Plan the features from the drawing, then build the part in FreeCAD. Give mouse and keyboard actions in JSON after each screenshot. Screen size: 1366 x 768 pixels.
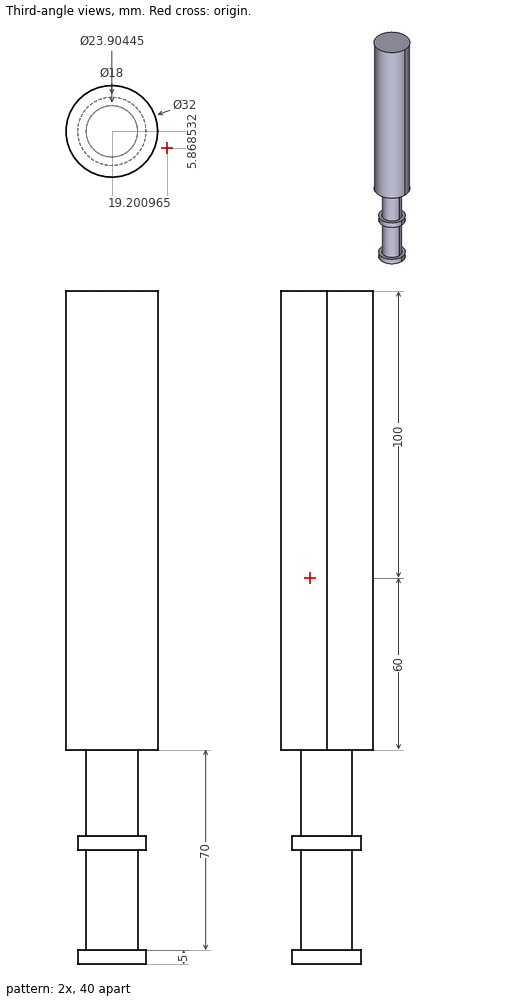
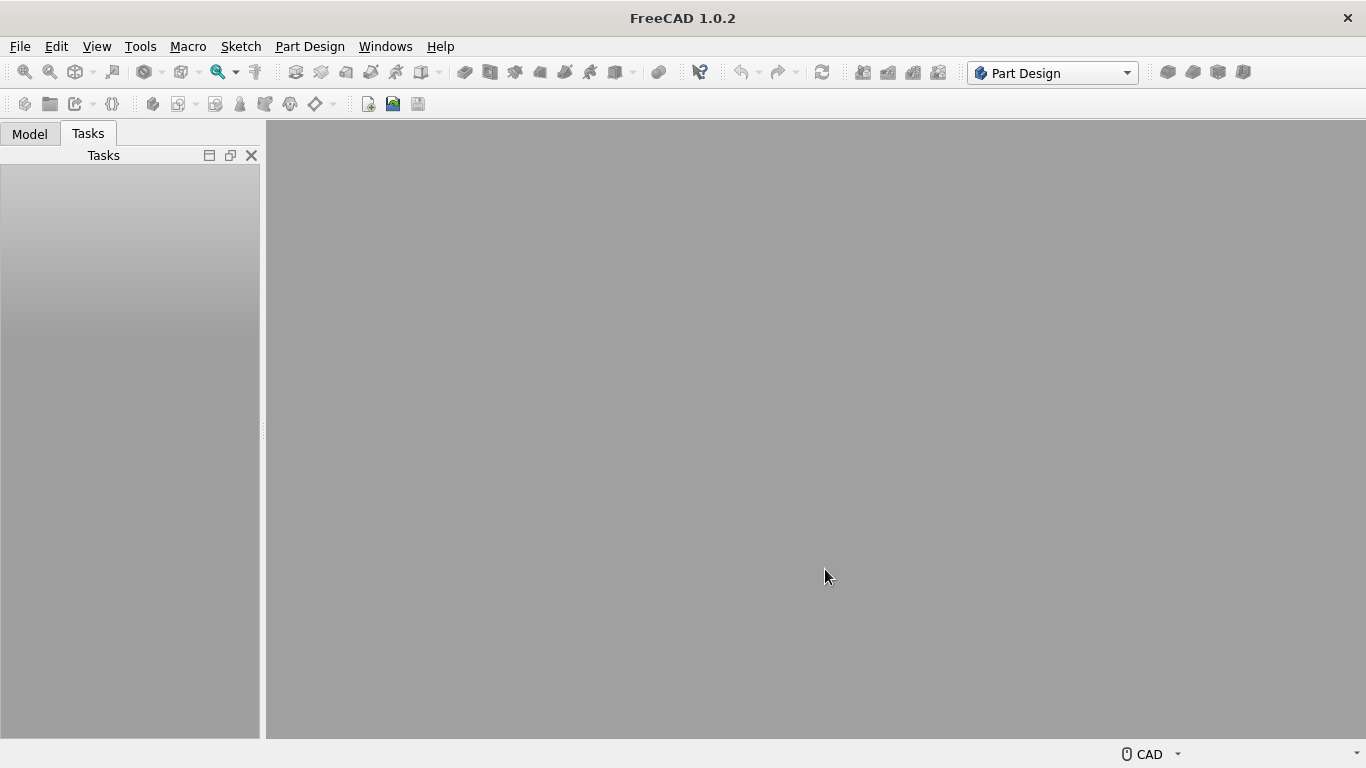
{"action": "key", "text": "ctrl+n"}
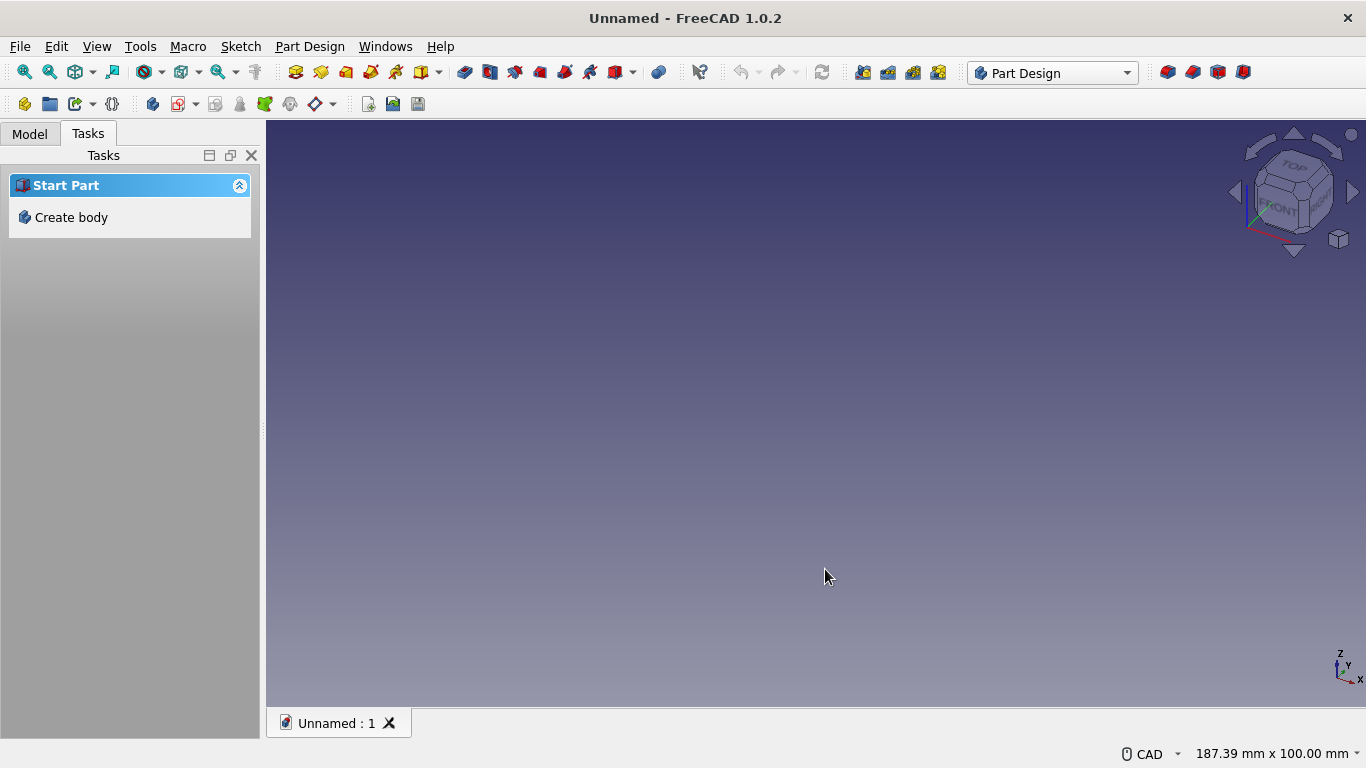
{"action": "left_click", "coordinate": [178, 104]}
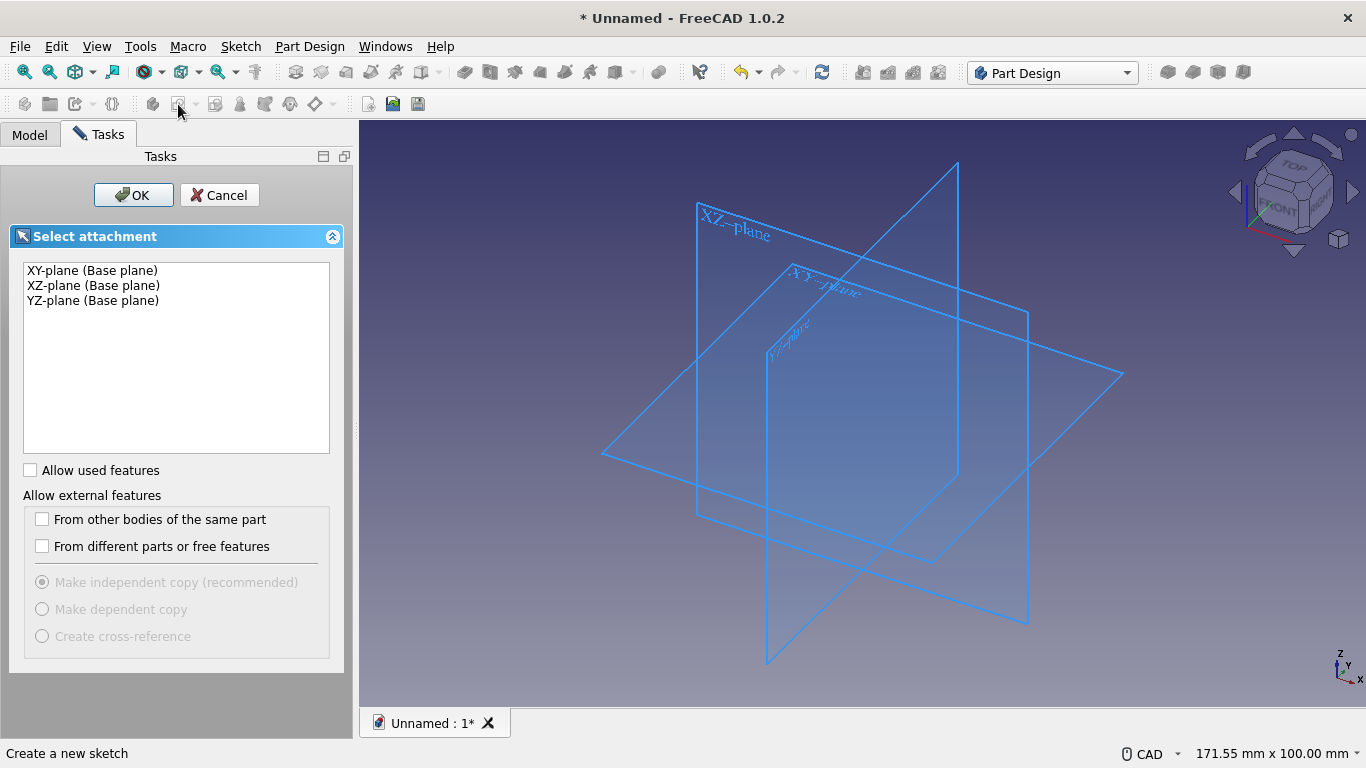
{"action": "left_click", "coordinate": [84, 270]}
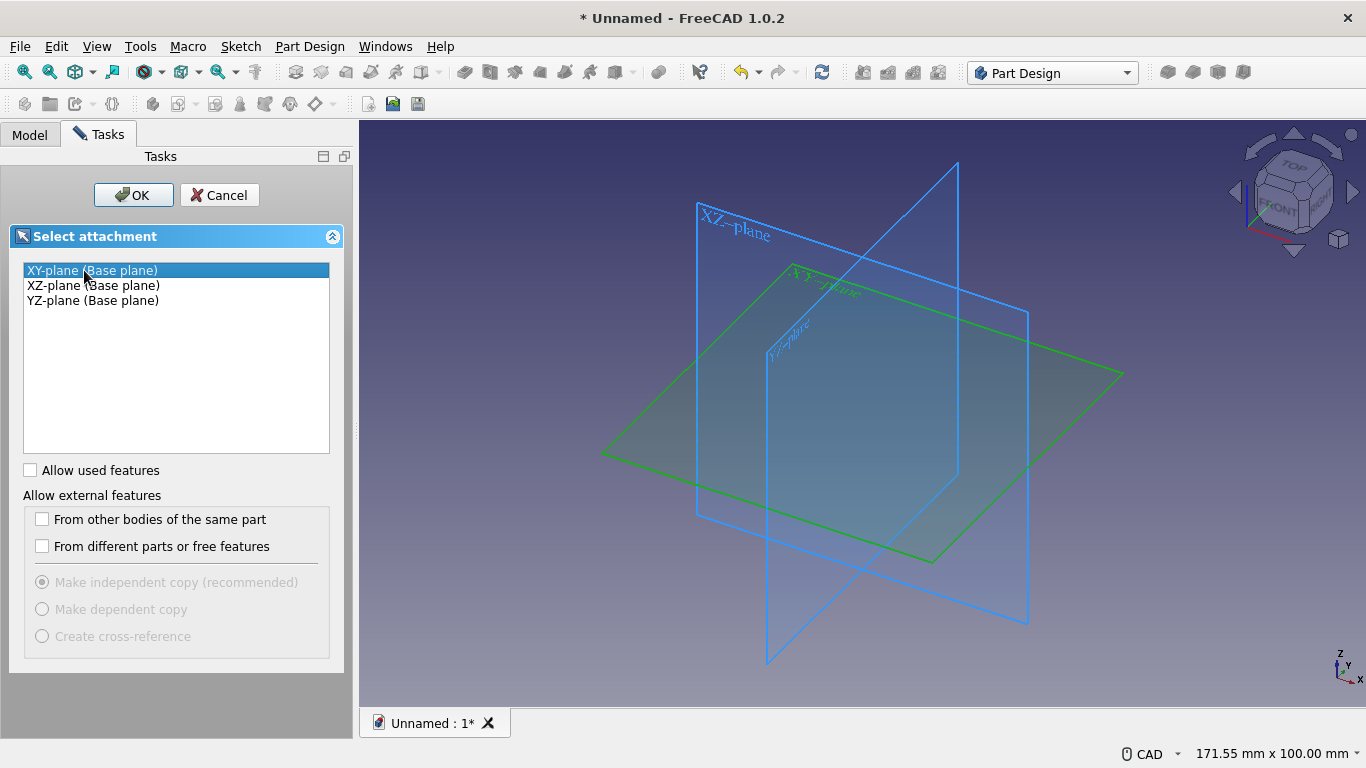
{"action": "left_click", "coordinate": [134, 195]}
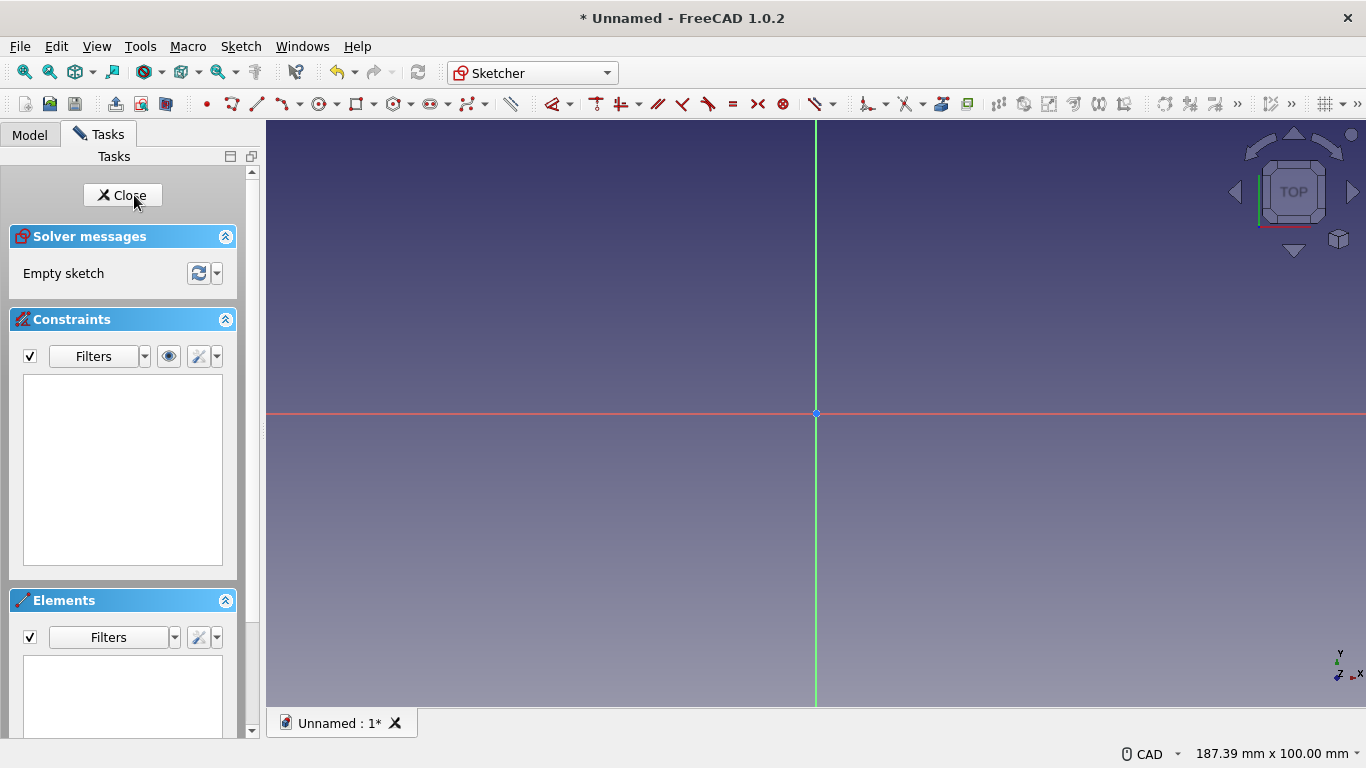
{"action": "scroll", "coordinate": [670, 337], "scroll_direction": "up", "scroll_amount": 3}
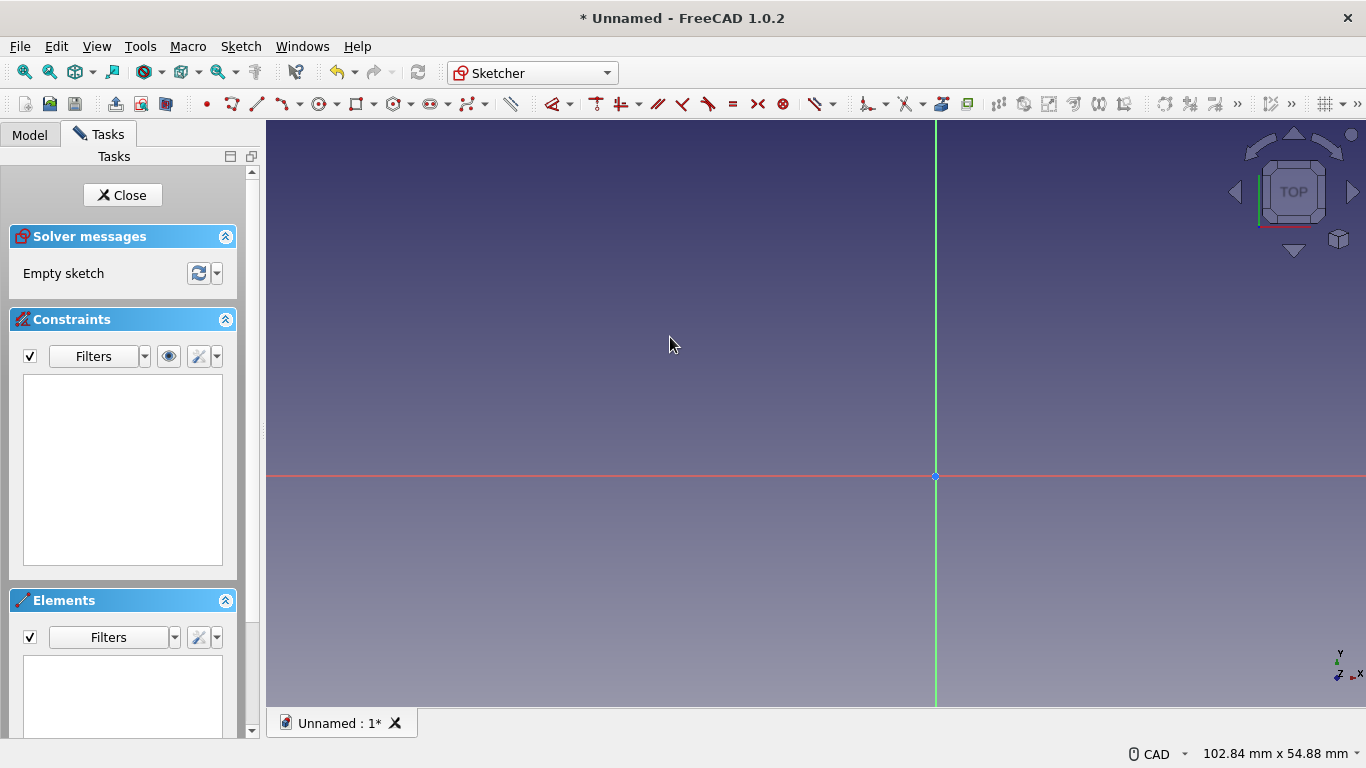
{"action": "left_click", "coordinate": [318, 104]}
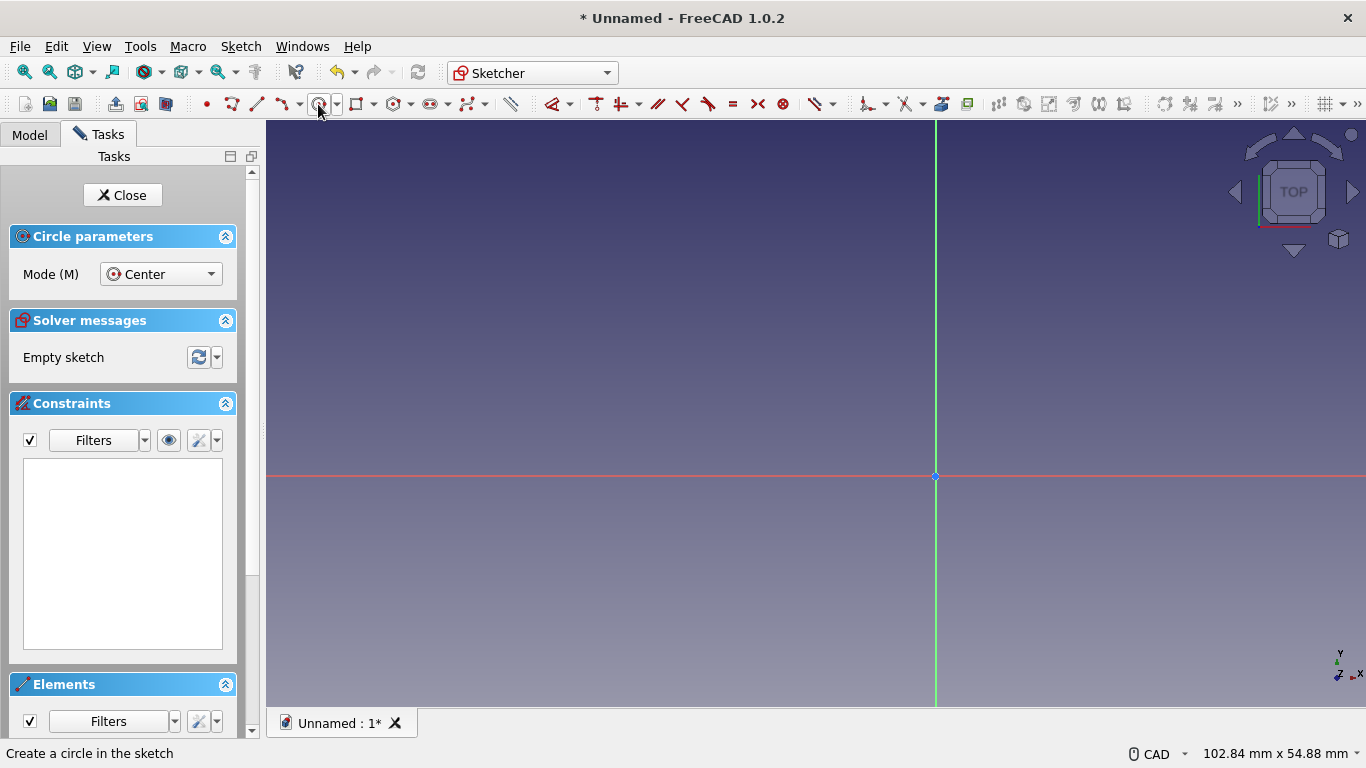
{"action": "left_click", "coordinate": [730, 413]}
{"action": "mouse_move", "coordinate": [851, 292]}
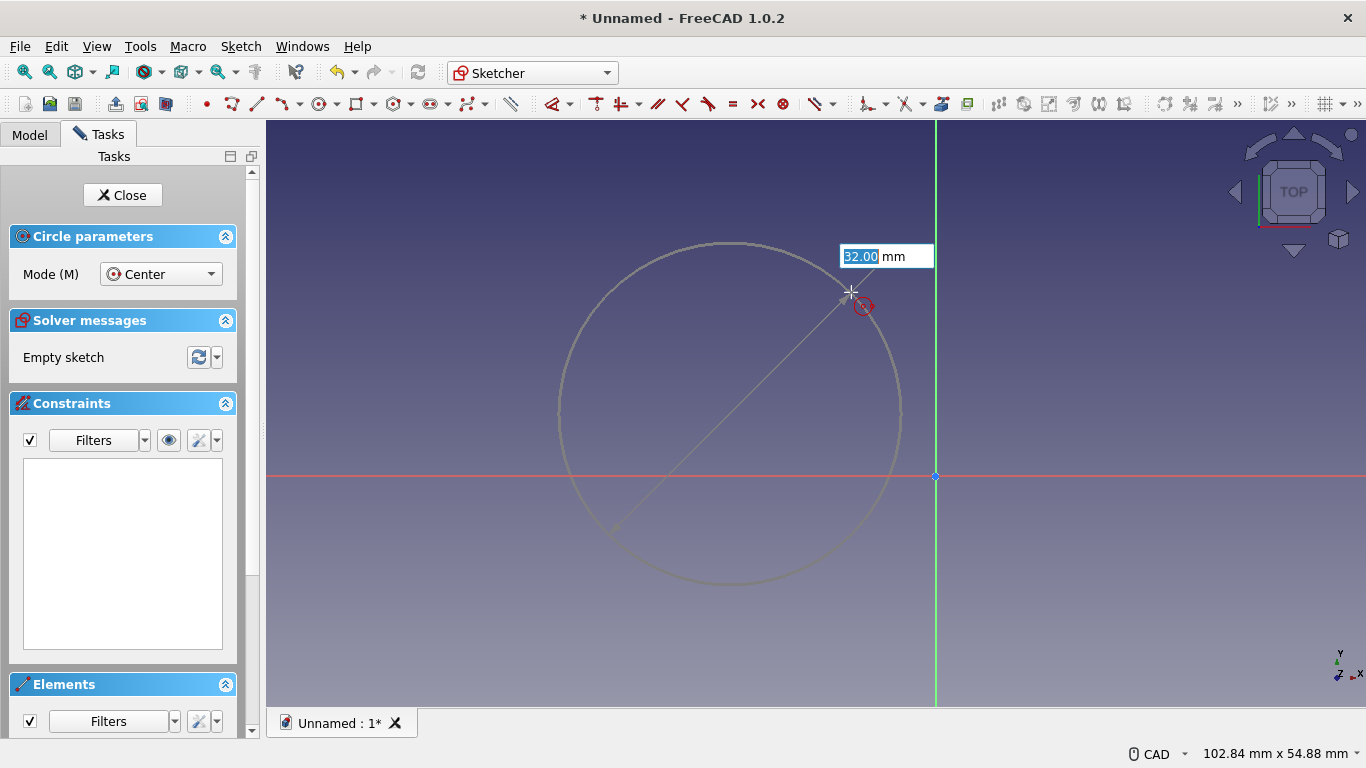
{"action": "type", "text": "32"}
{"action": "key", "text": "Return"}
{"action": "key", "text": "Escape"}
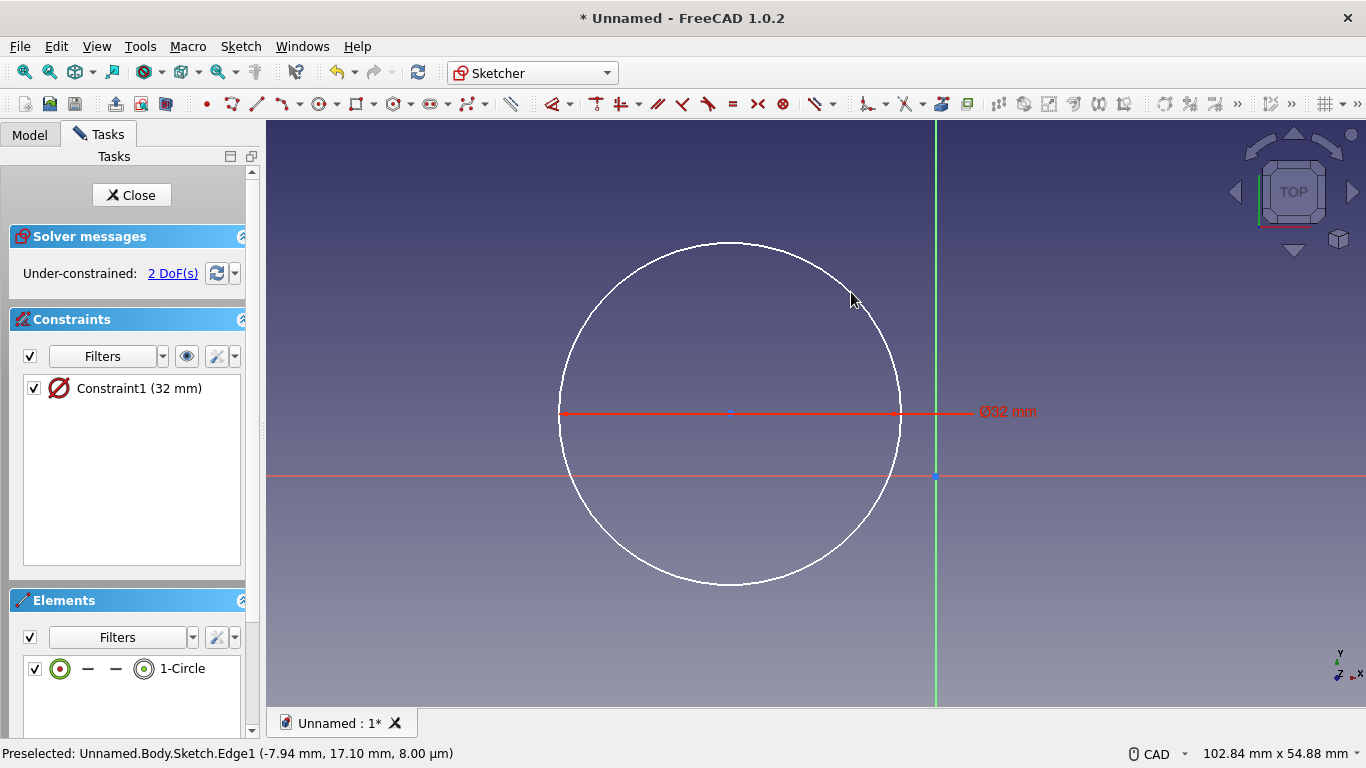
{"action": "key", "text": "d"}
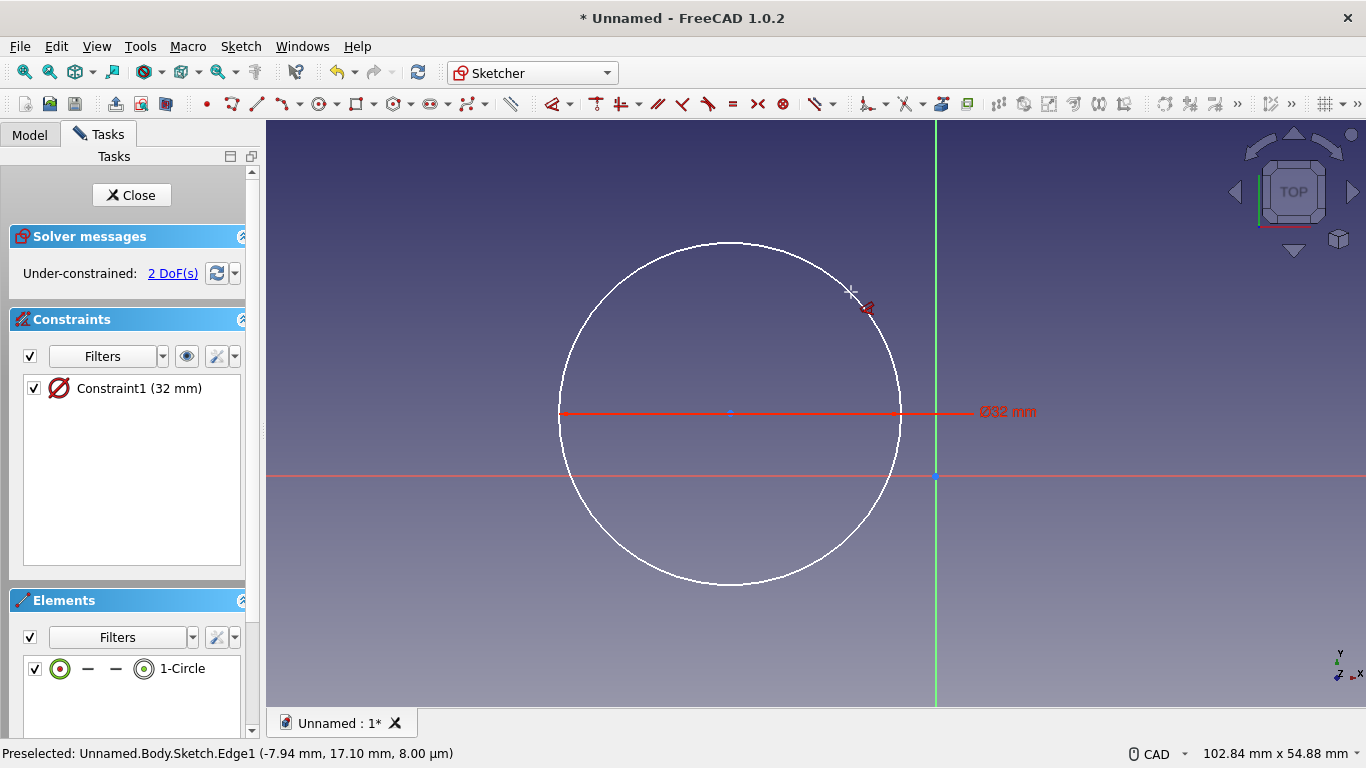
{"action": "left_click", "coordinate": [730, 414]}
{"action": "left_click", "coordinate": [970, 445]}